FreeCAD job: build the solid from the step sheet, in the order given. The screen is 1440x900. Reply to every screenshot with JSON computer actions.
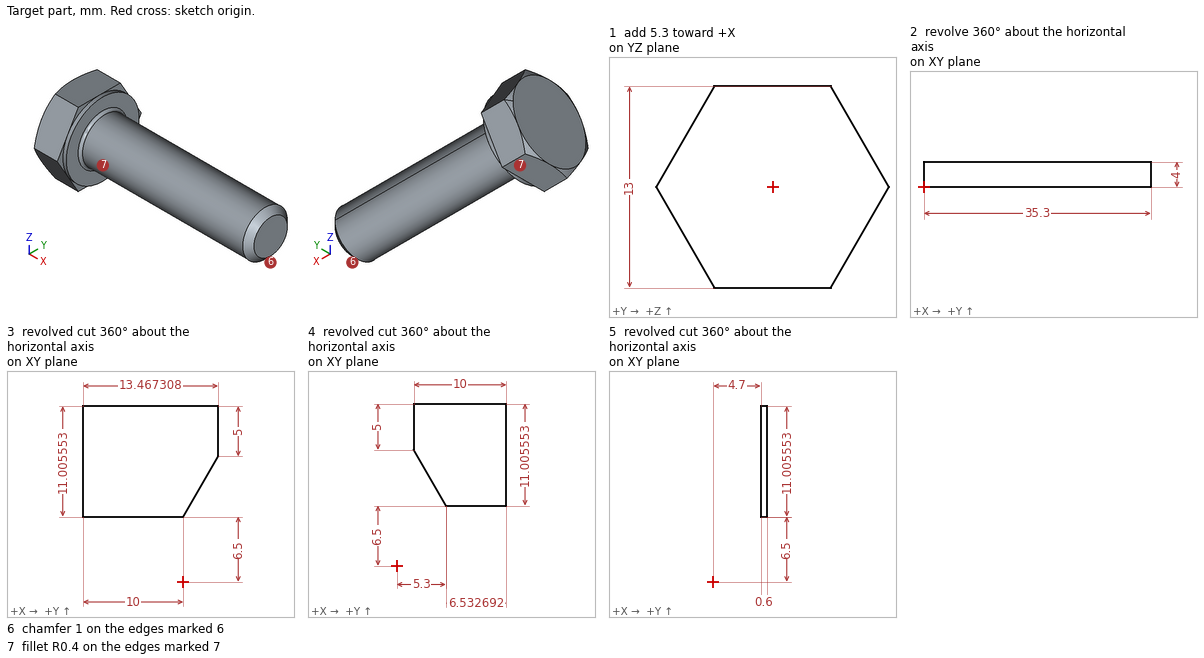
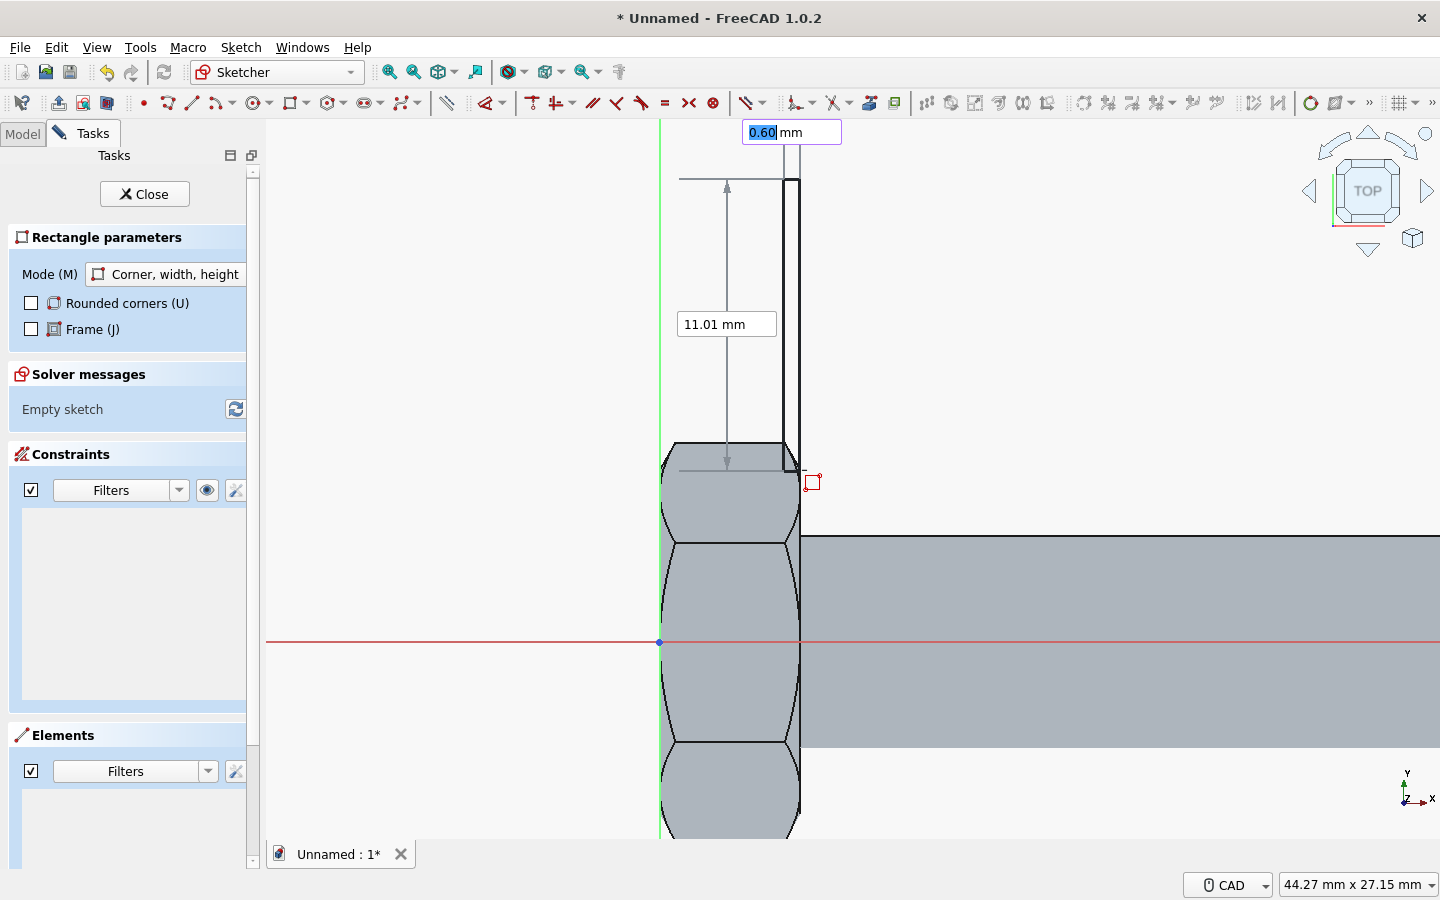
{"action": "type", "text": "0.6"}
{"action": "key", "text": "Tab"}
{"action": "type", "text": "11.005553"}
{"action": "key", "text": "Return"}
{"action": "key", "text": "Escape"}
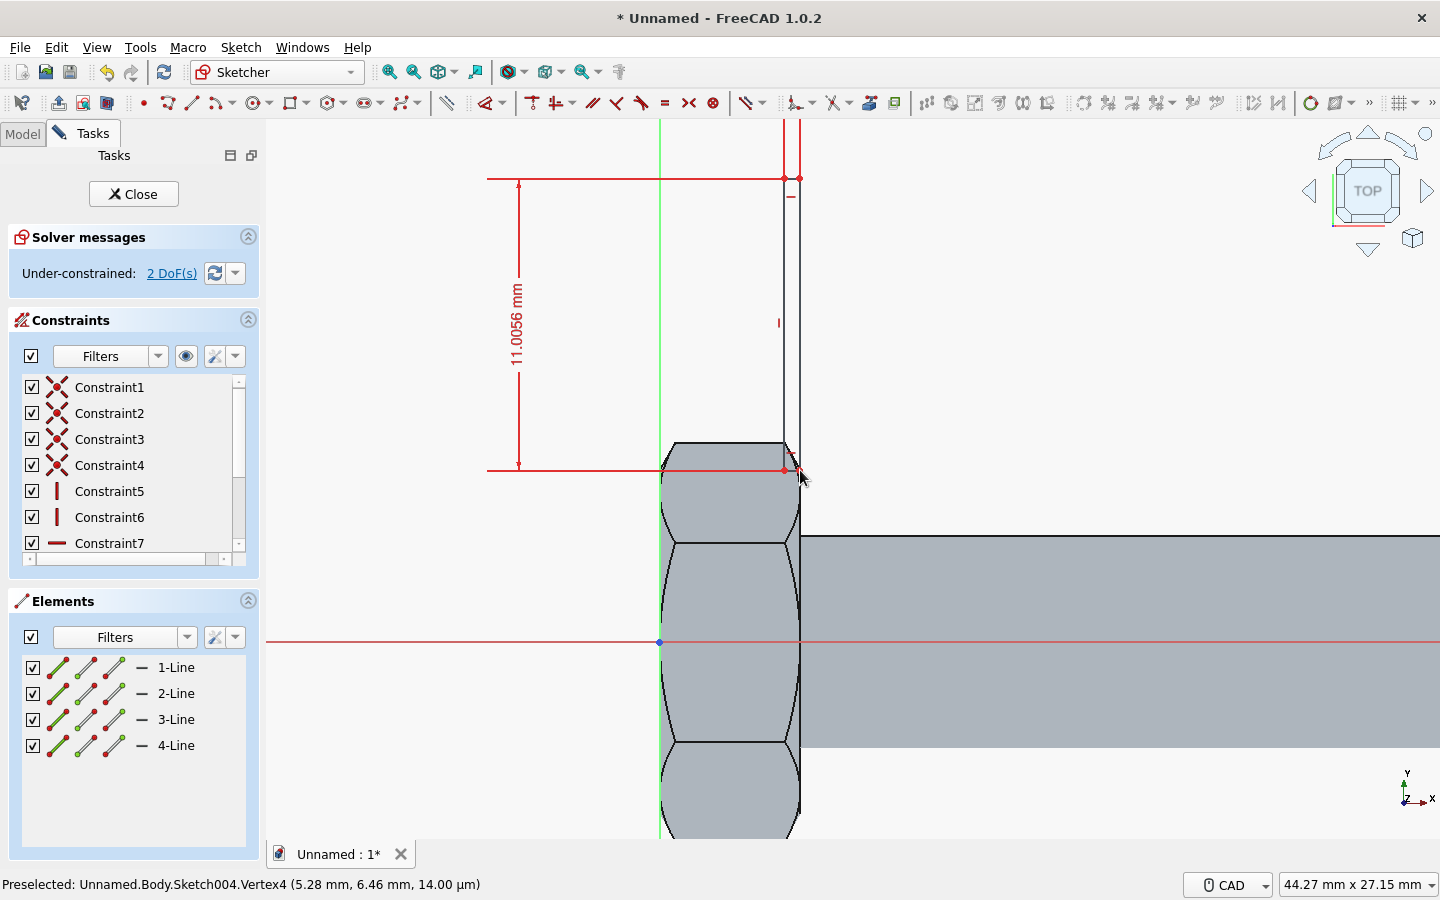
{"action": "key", "text": "d"}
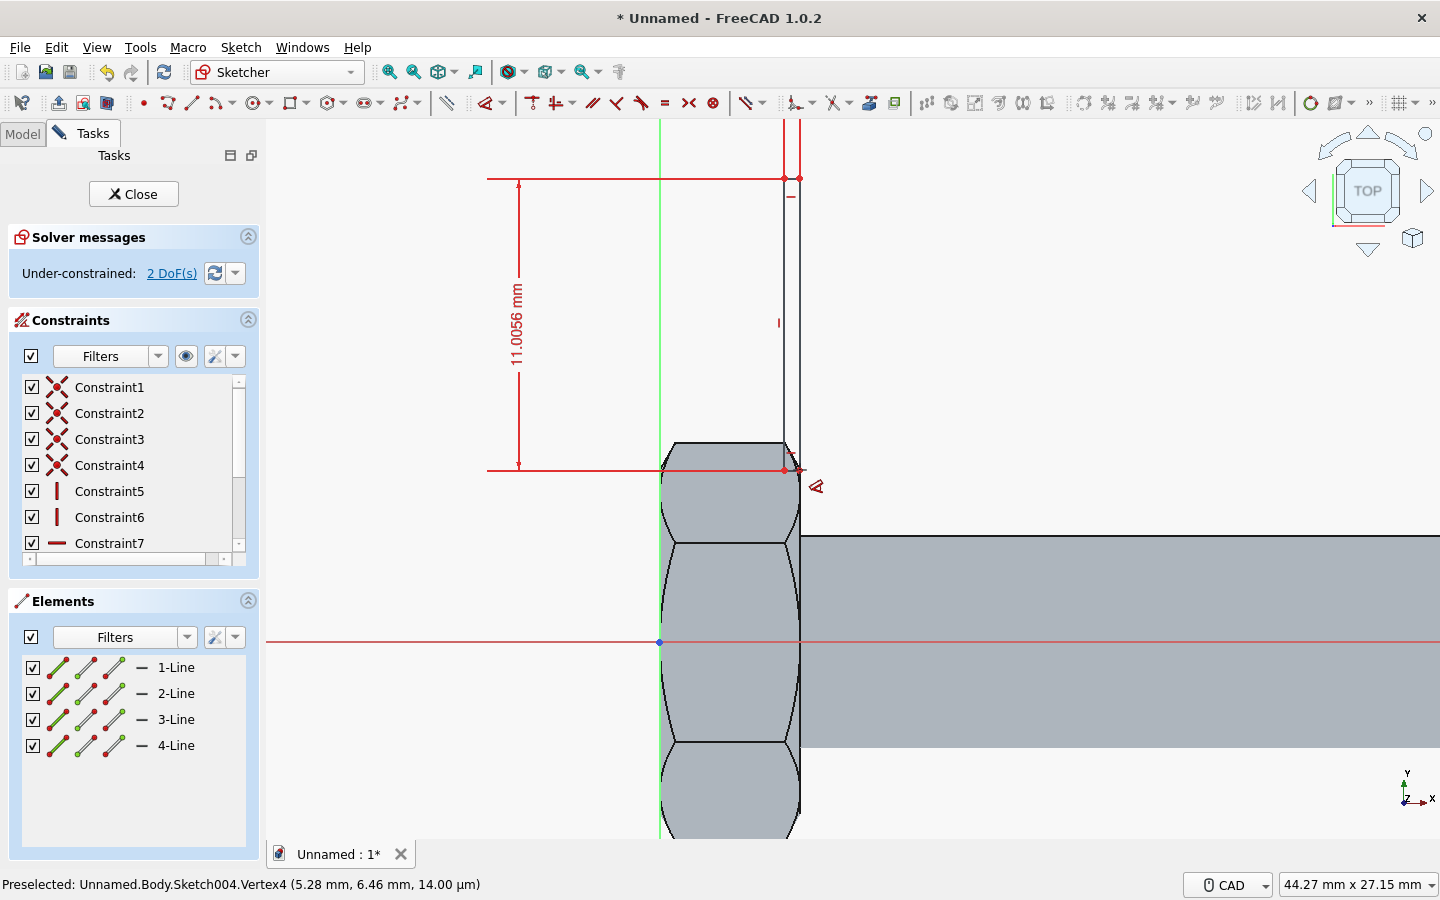
{"action": "left_click", "coordinate": [784, 179]}
{"action": "left_click", "coordinate": [722, 676]}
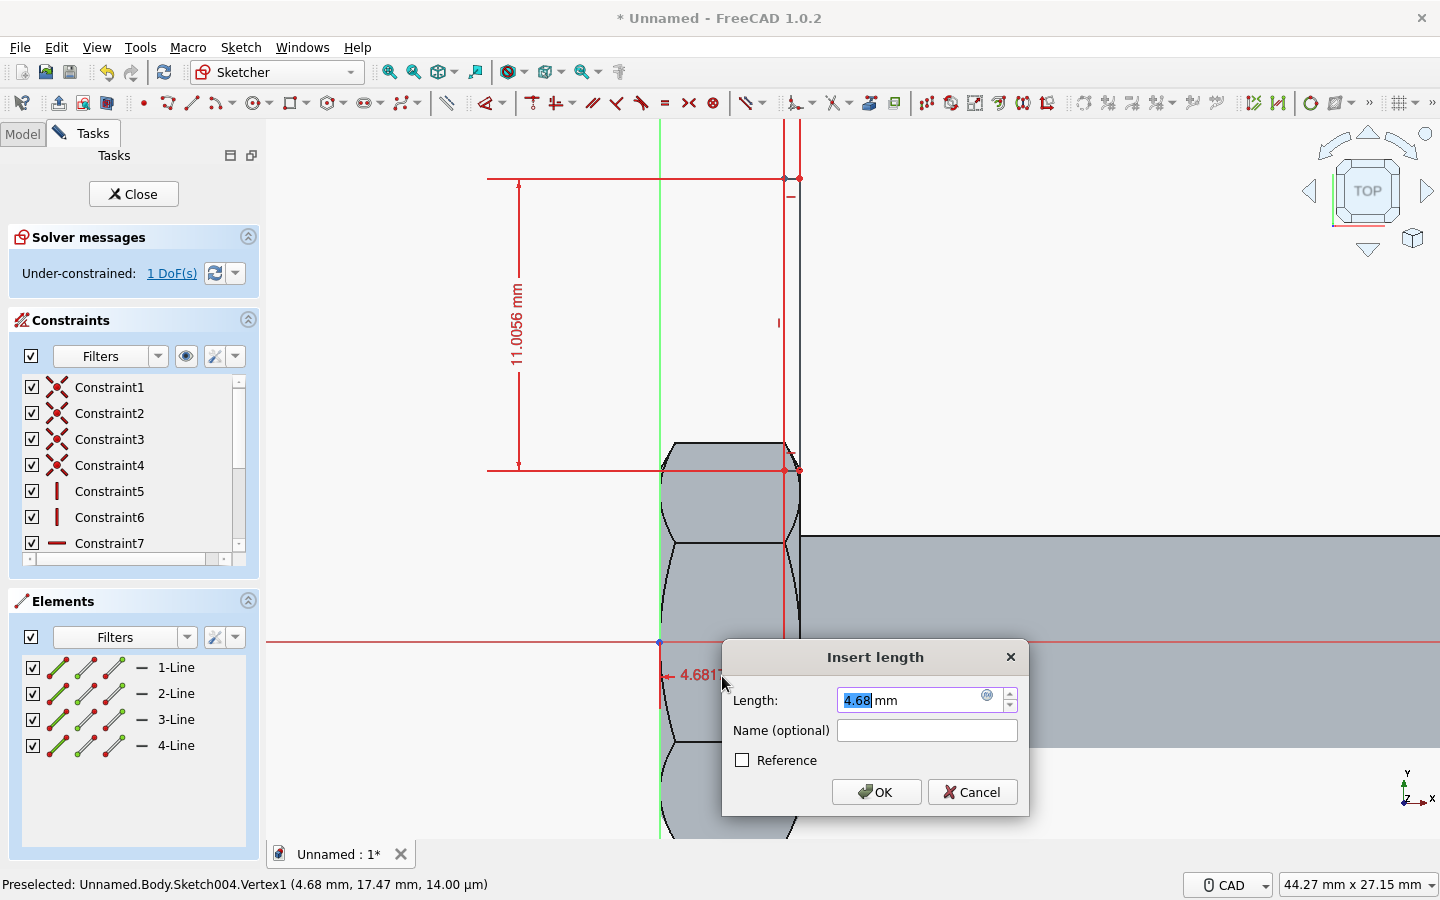
{"action": "type", "text": "4.7"}
{"action": "key", "text": "Return"}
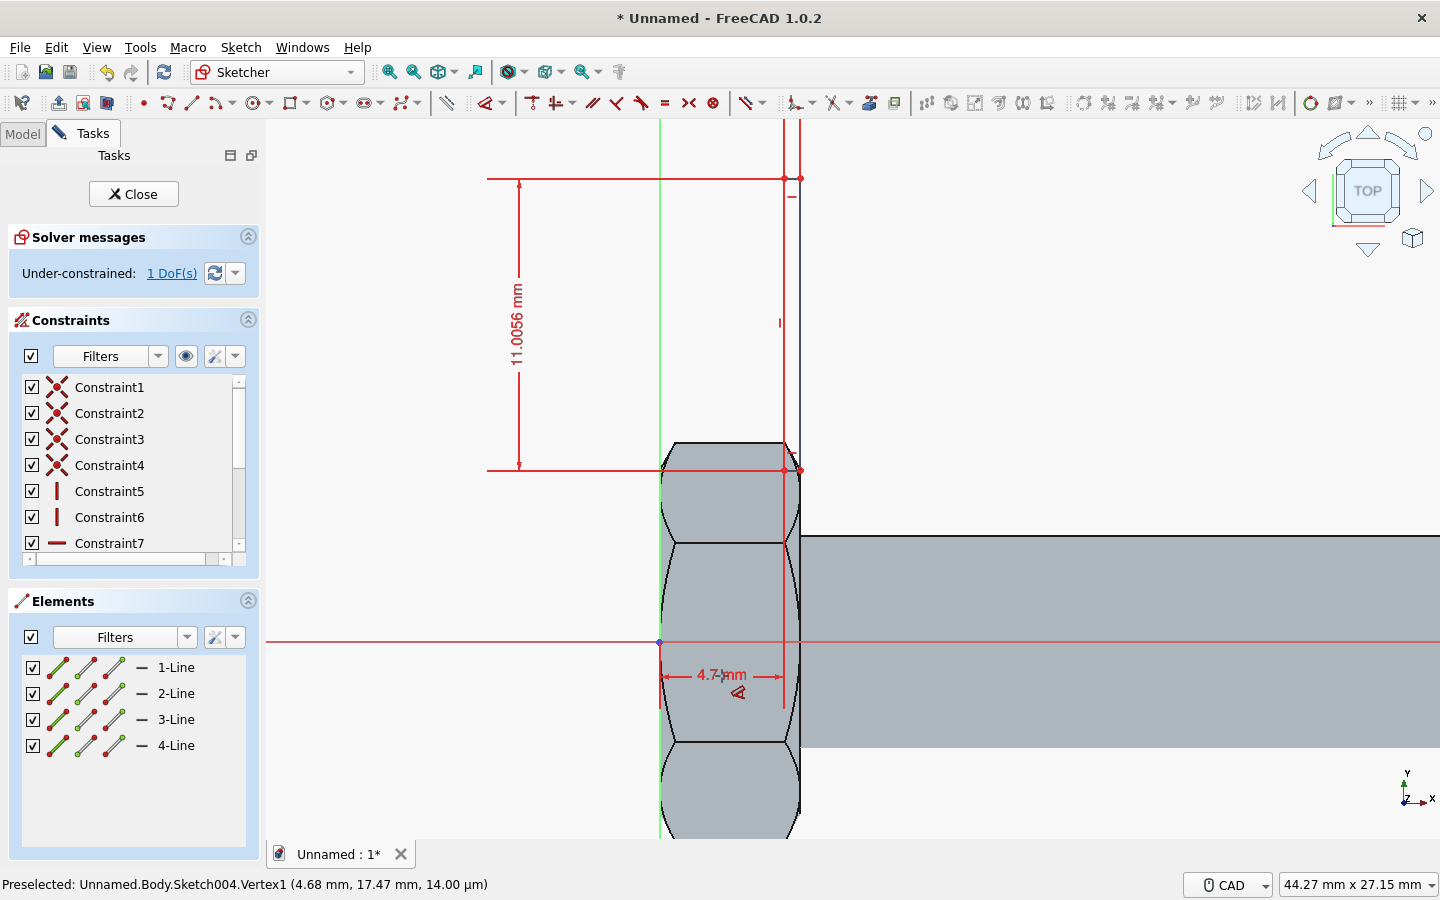
{"action": "left_click", "coordinate": [784, 471]}
{"action": "left_click", "coordinate": [626, 557]}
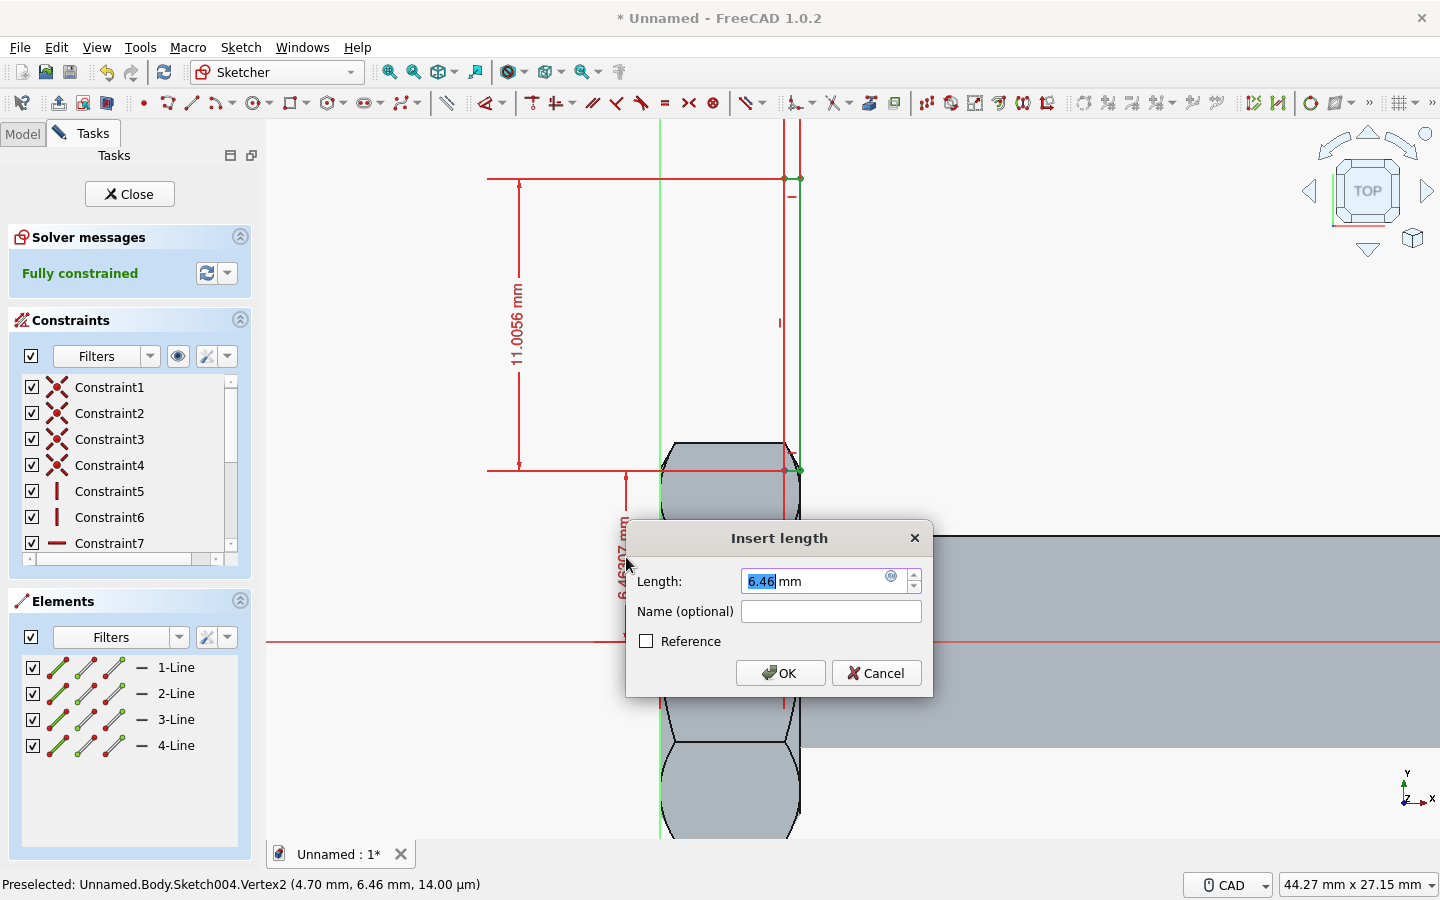
{"action": "type", "text": "6.5"}
{"action": "key", "text": "Return"}
{"action": "key", "text": "Escape"}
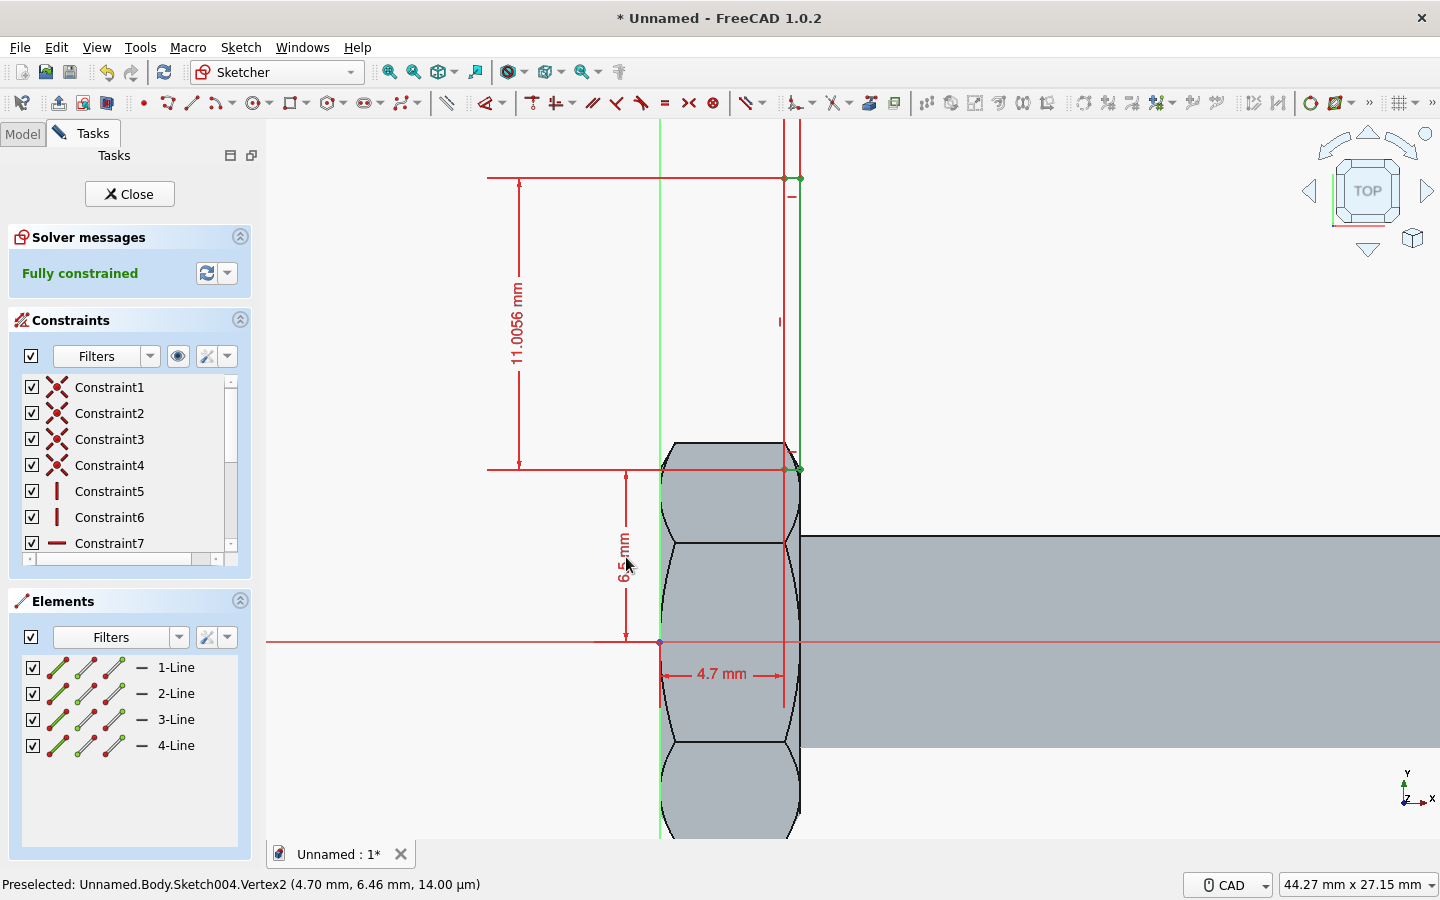
{"action": "left_click", "coordinate": [130, 194]}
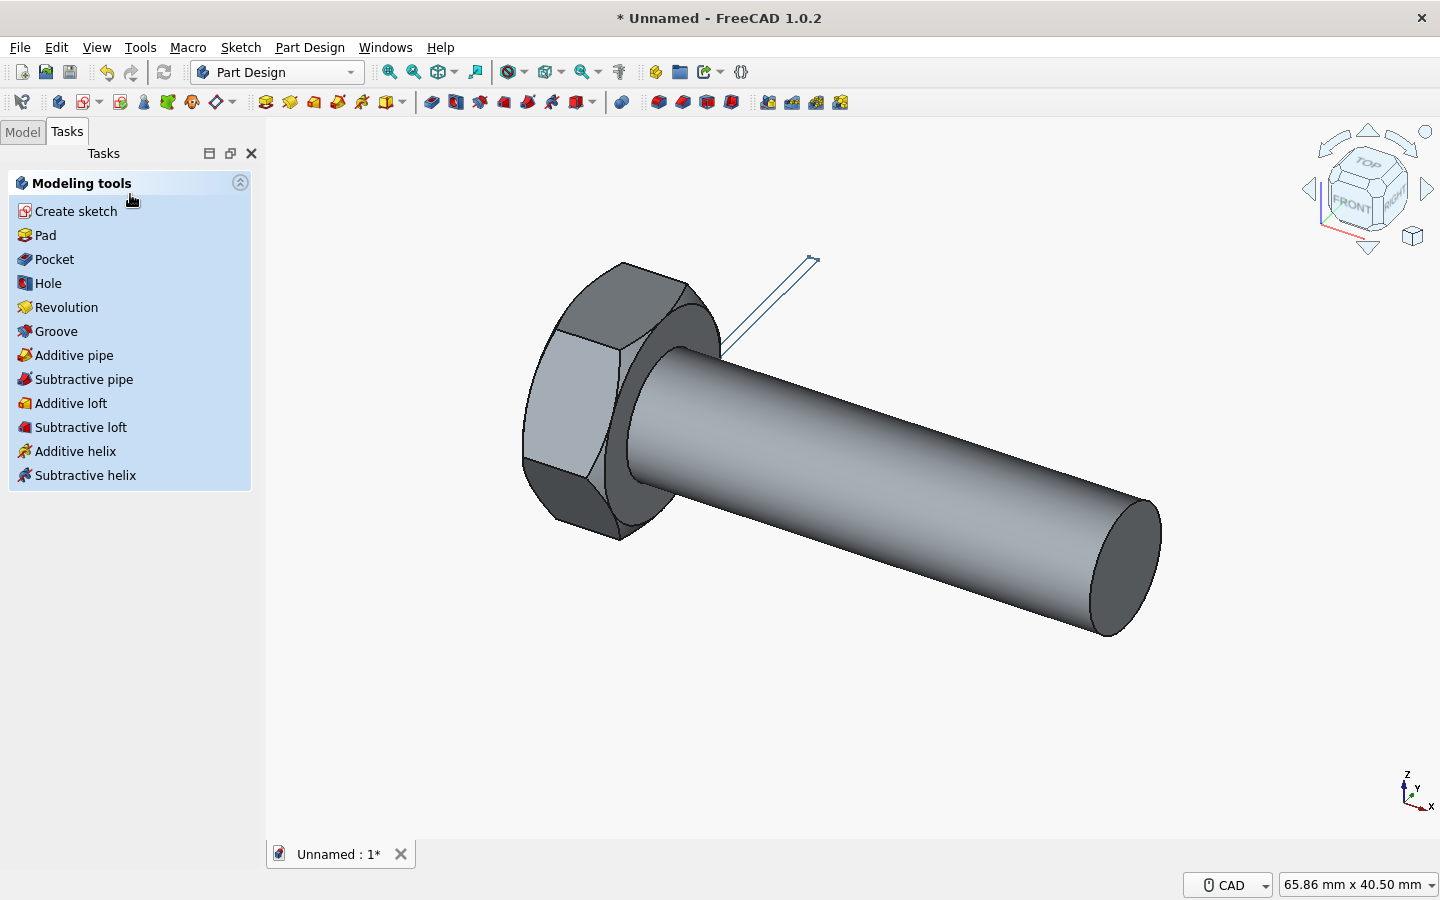
{"action": "left_click", "coordinate": [480, 102]}